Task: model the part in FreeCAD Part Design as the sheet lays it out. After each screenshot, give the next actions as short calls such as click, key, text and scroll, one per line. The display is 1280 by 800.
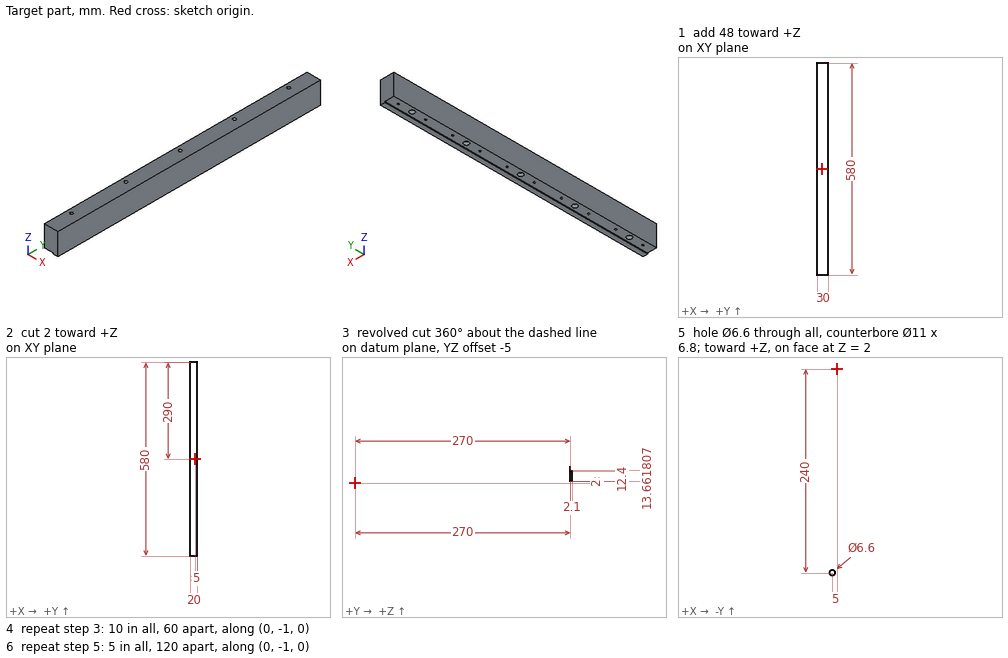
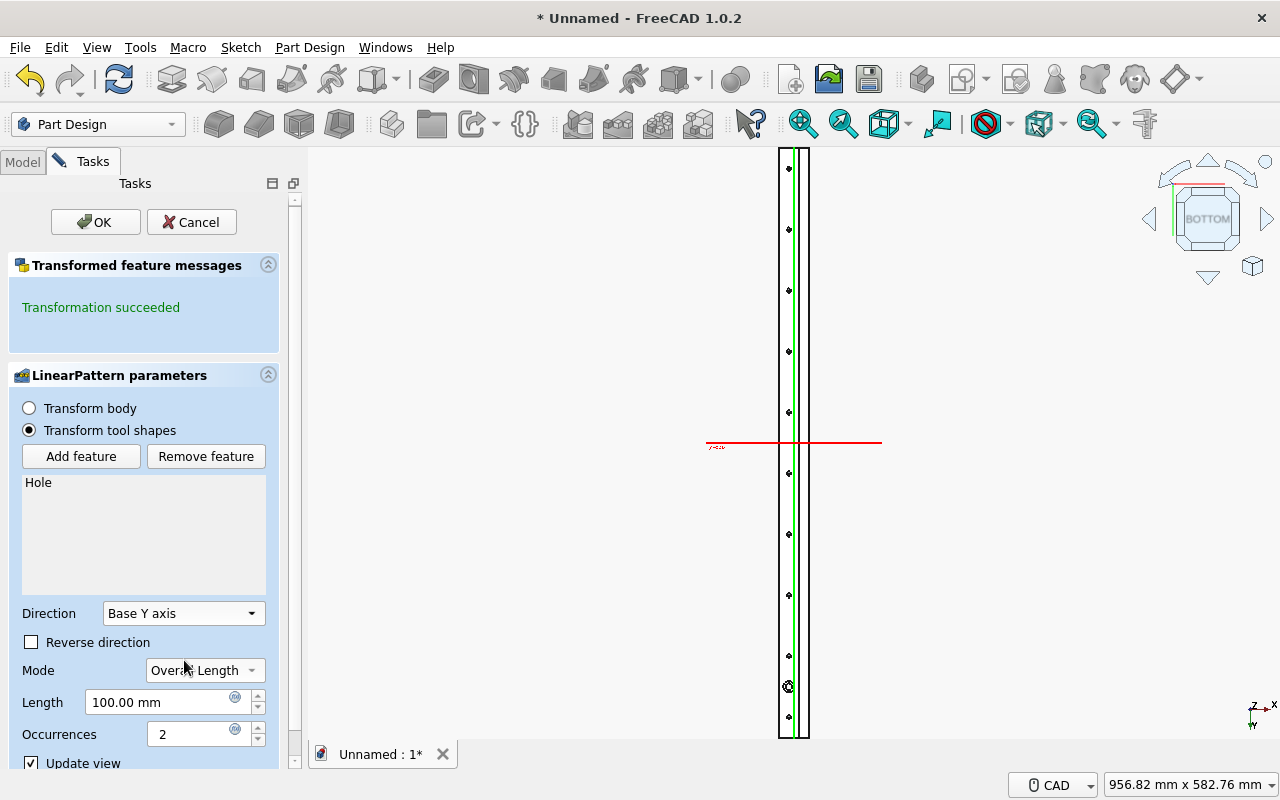
click(206, 670)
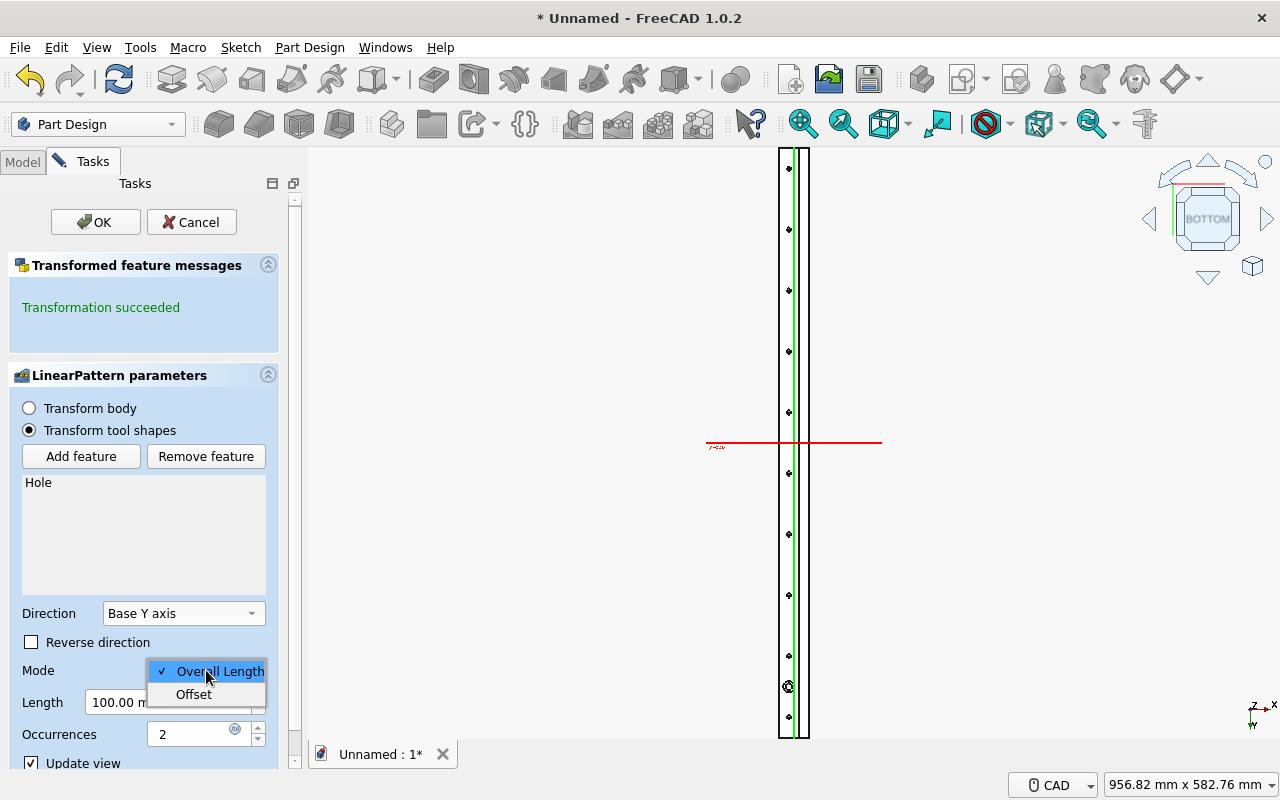
click(206, 694)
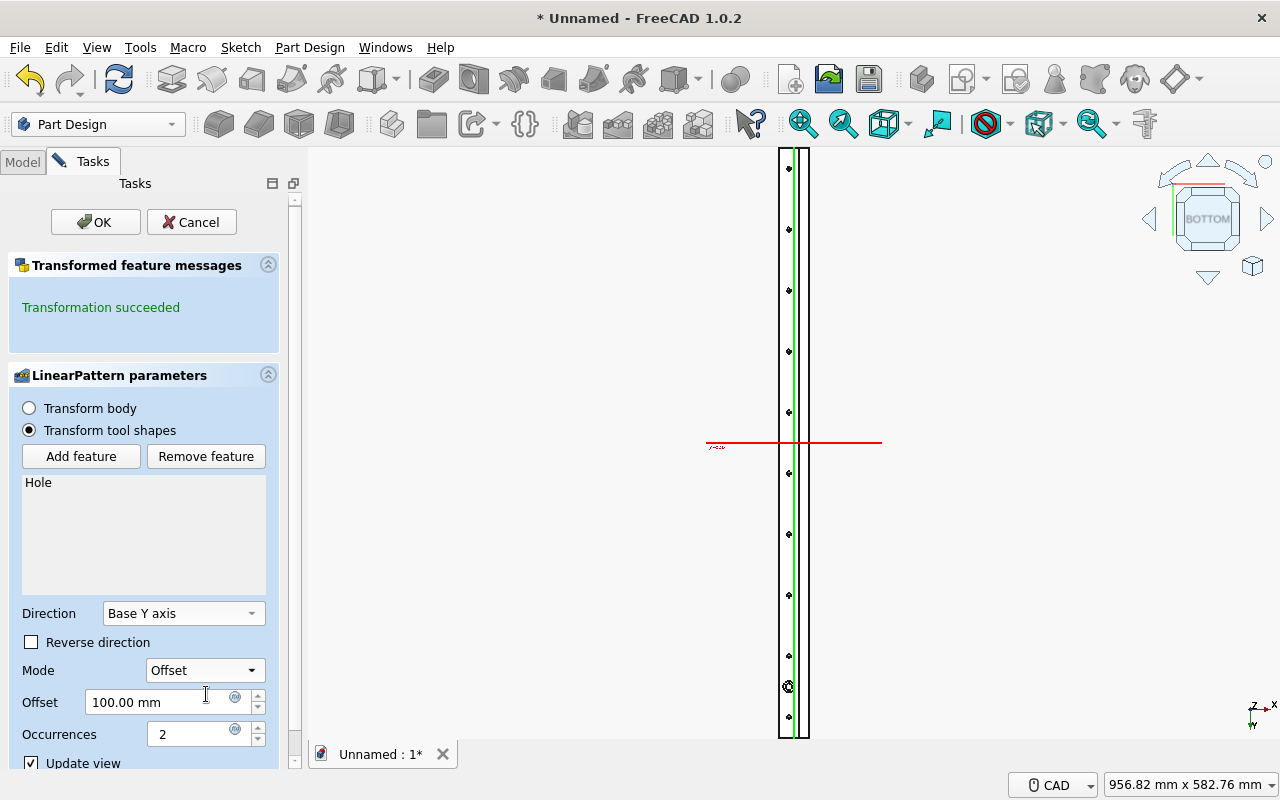
triple_click(168, 702)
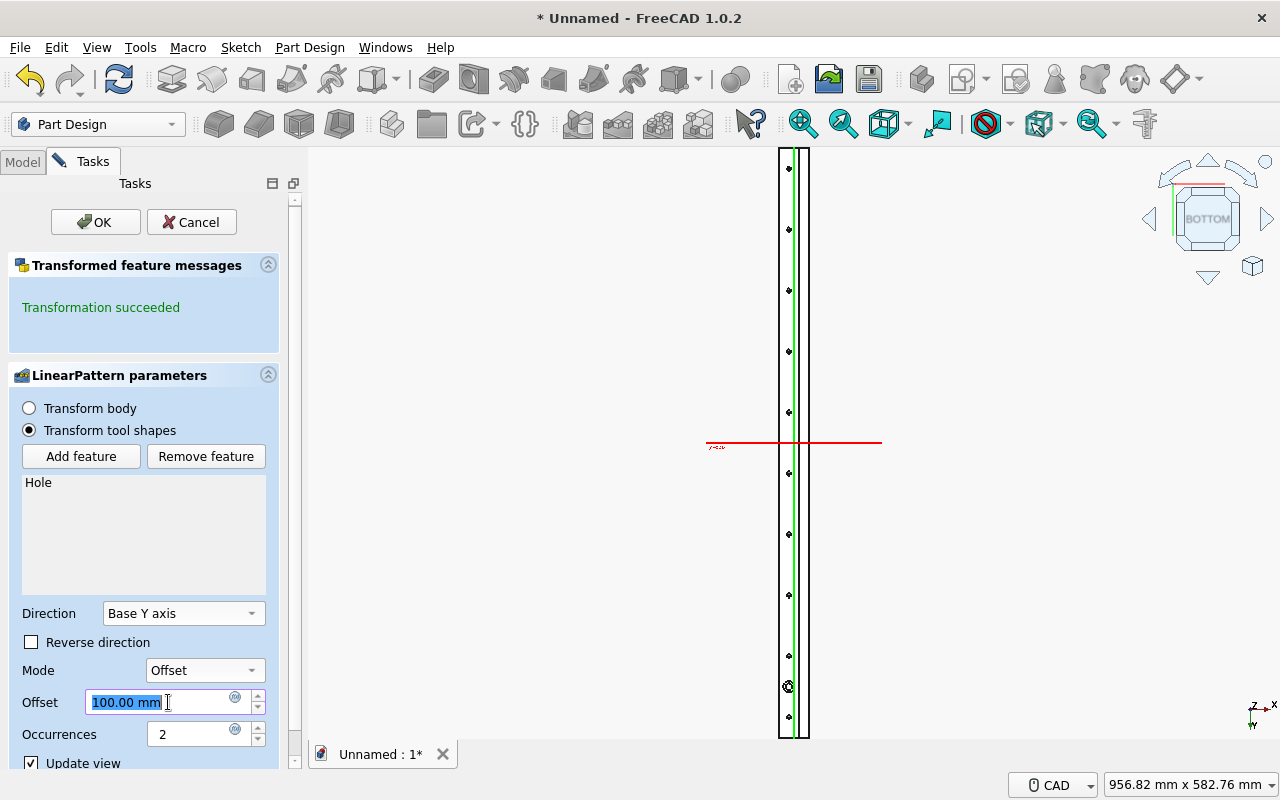
text(120)
key(Tab)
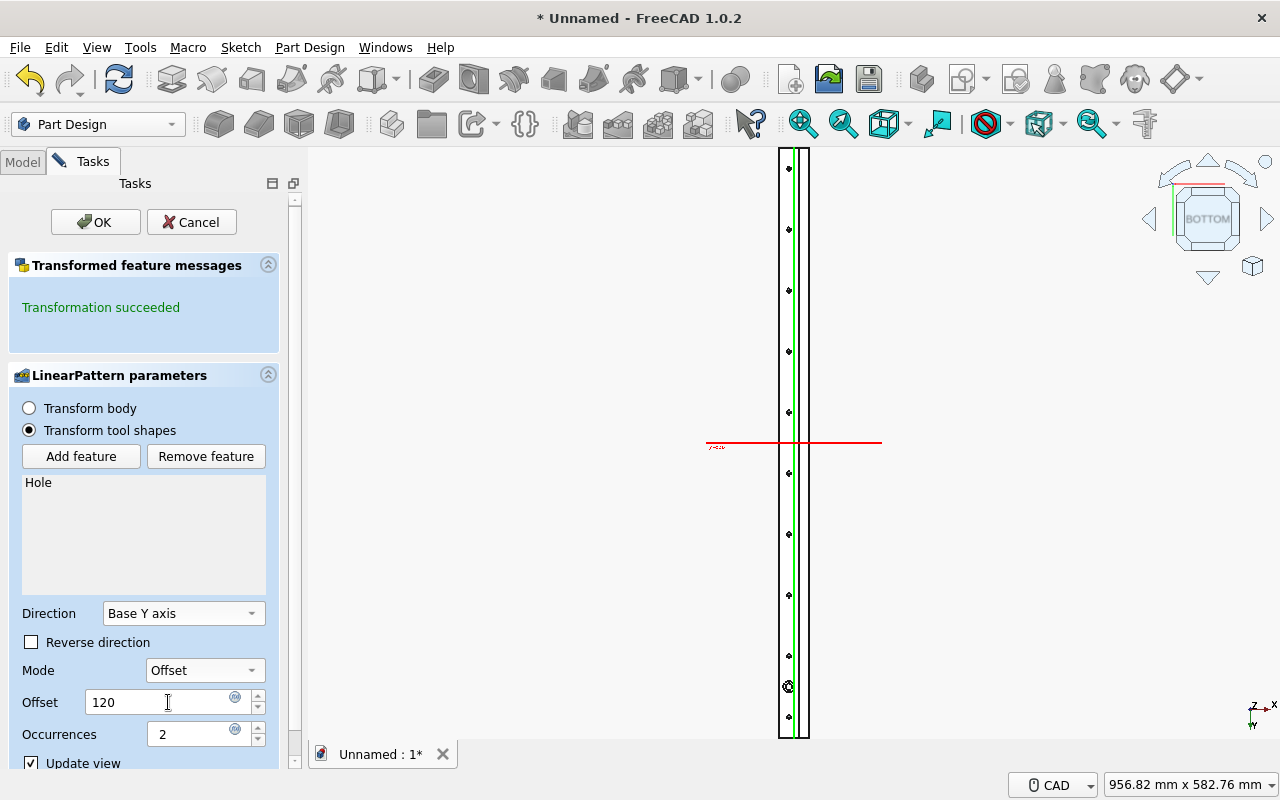
triple_click(198, 734)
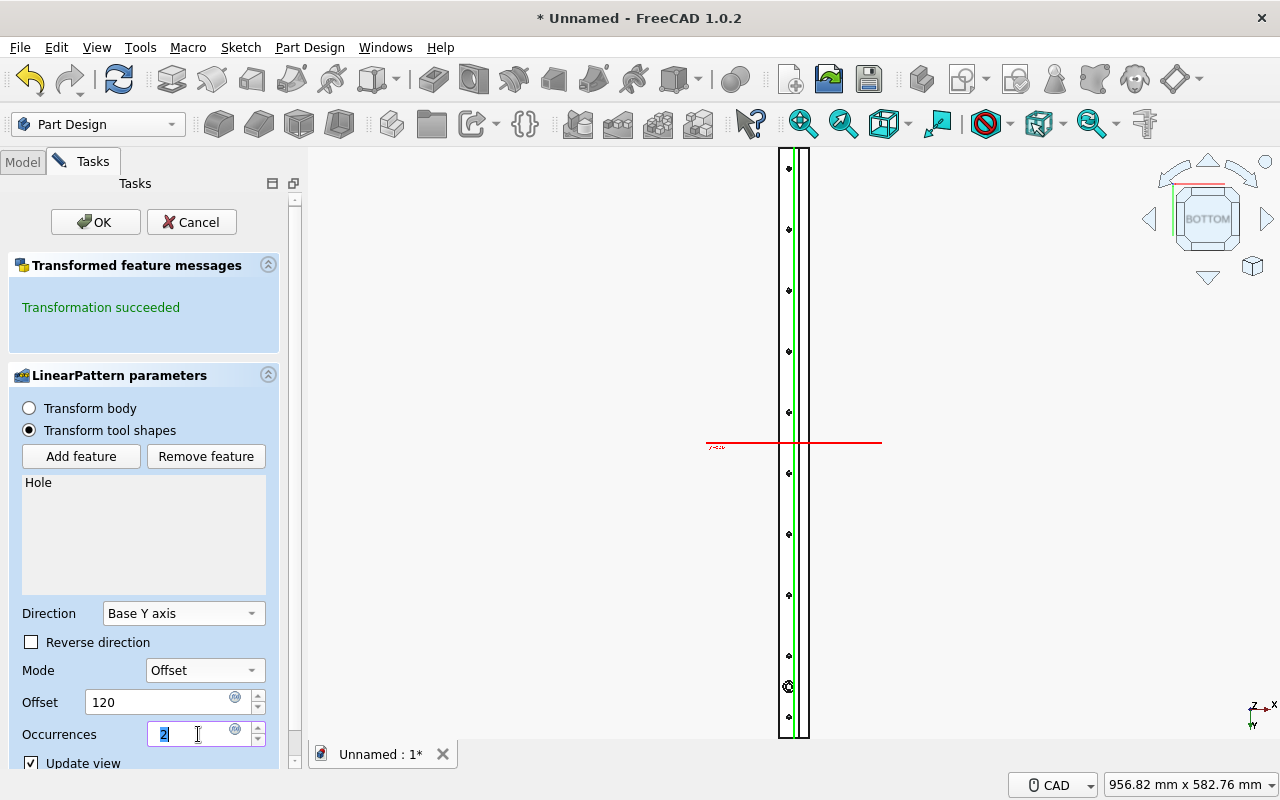
text(5)
key(Tab)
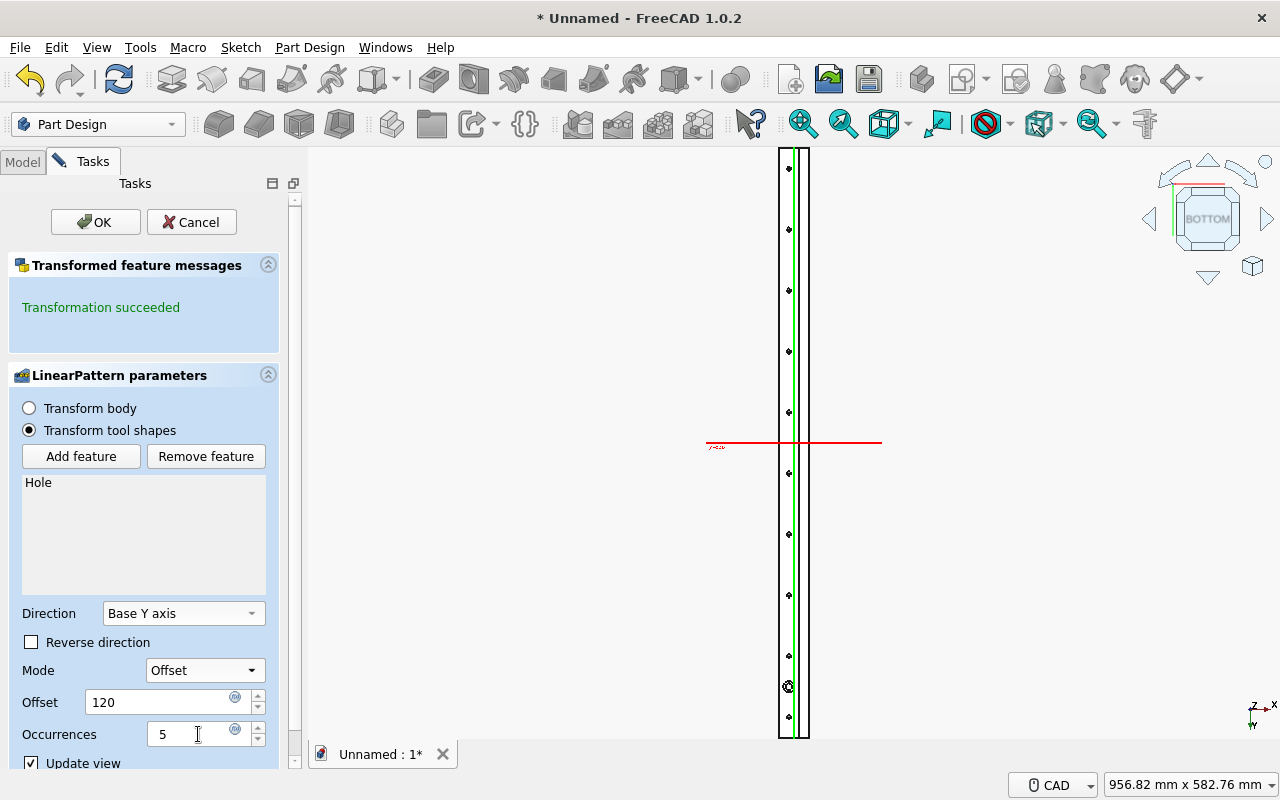
click(30, 642)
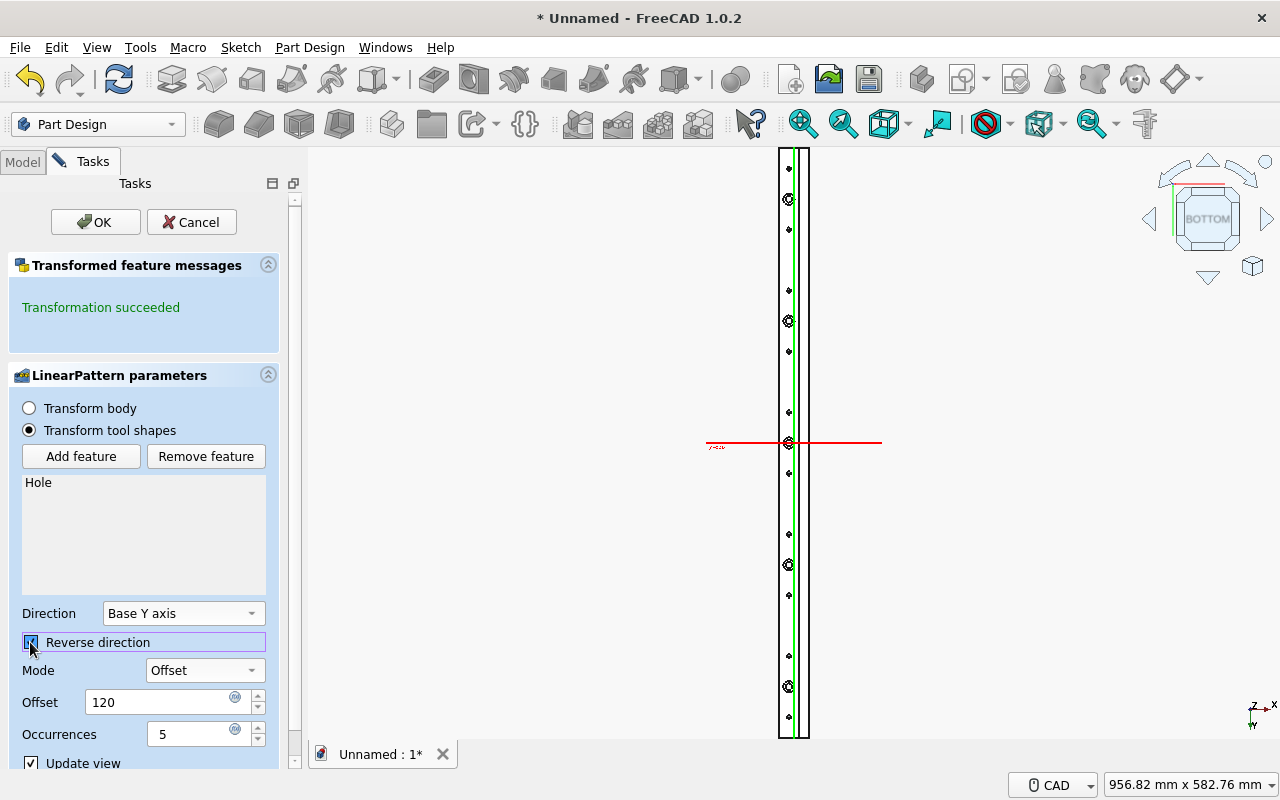
click(96, 222)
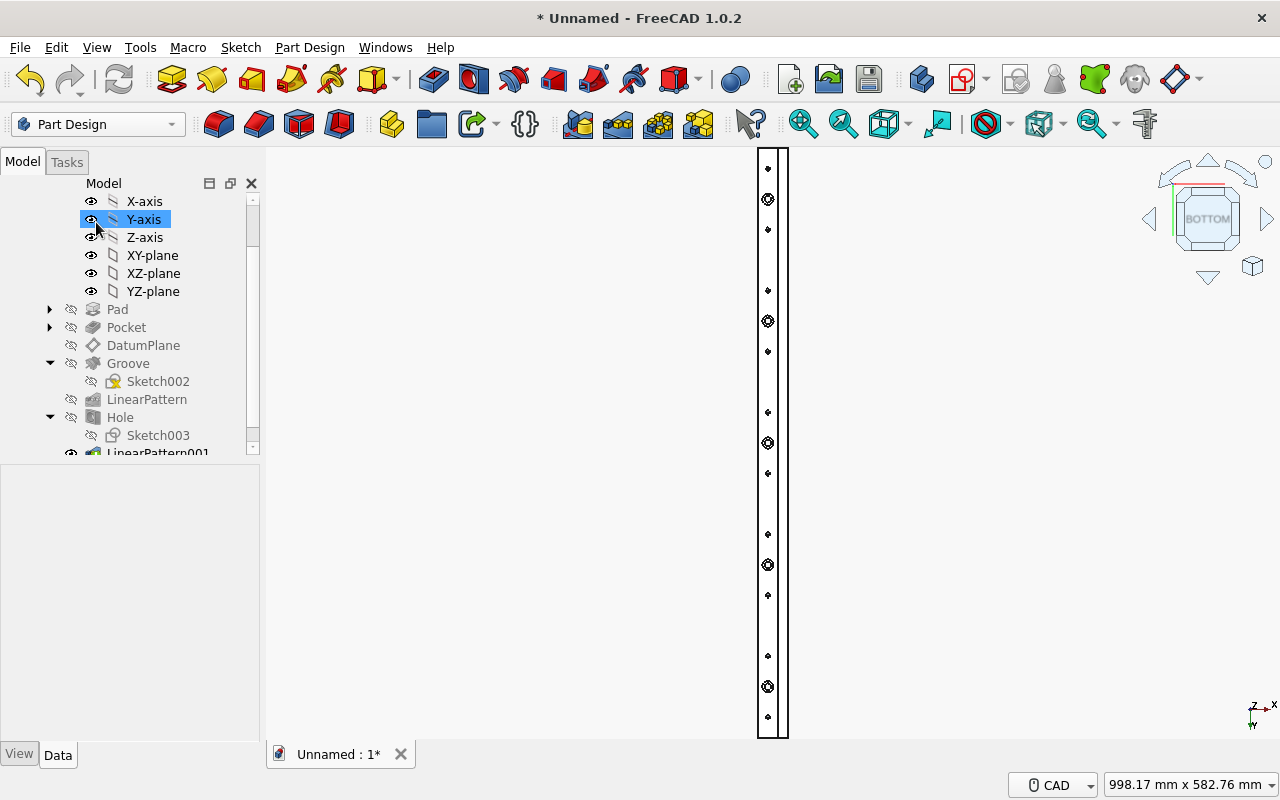
key(0)